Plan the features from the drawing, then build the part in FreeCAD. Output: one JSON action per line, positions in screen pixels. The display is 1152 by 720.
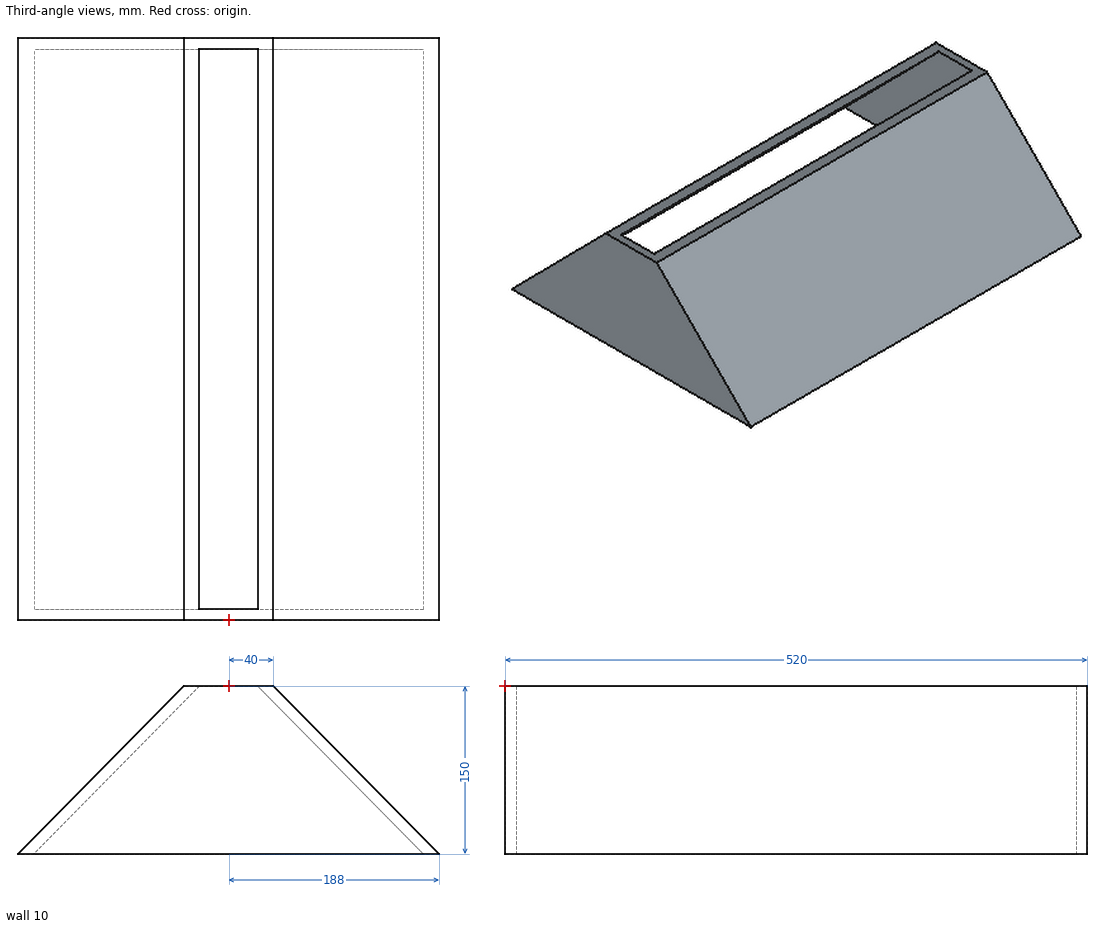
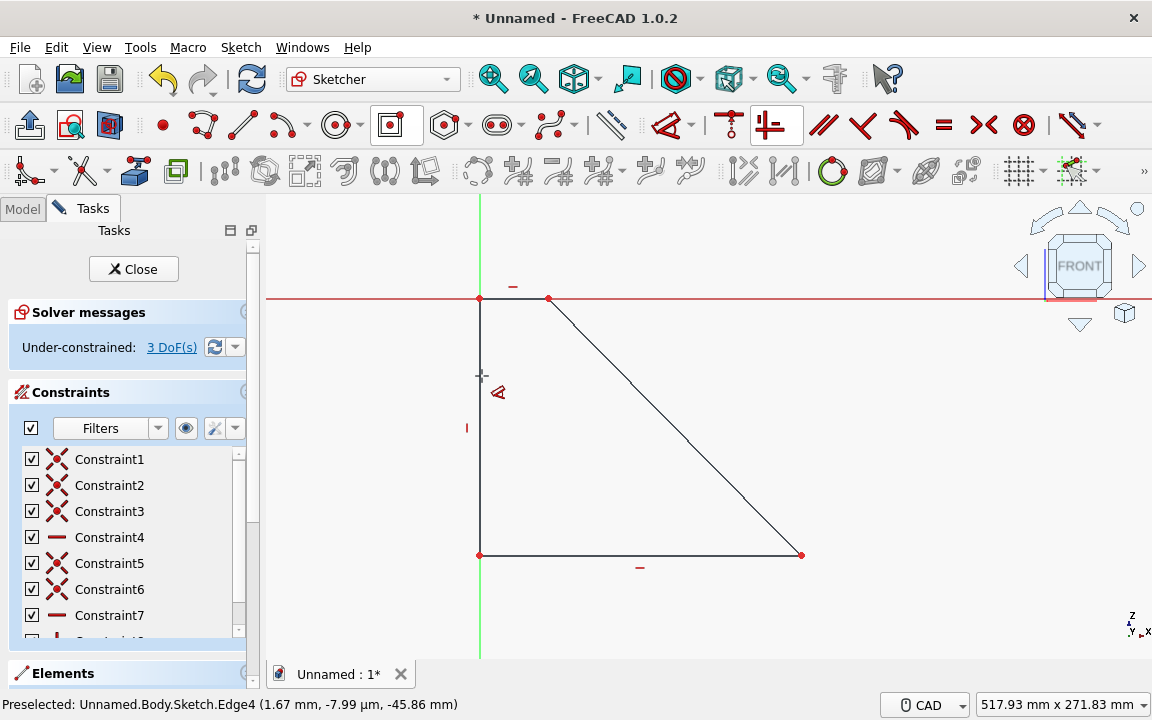
{"action": "left_click", "coordinate": [500, 299]}
{"action": "left_click", "coordinate": [514, 265]}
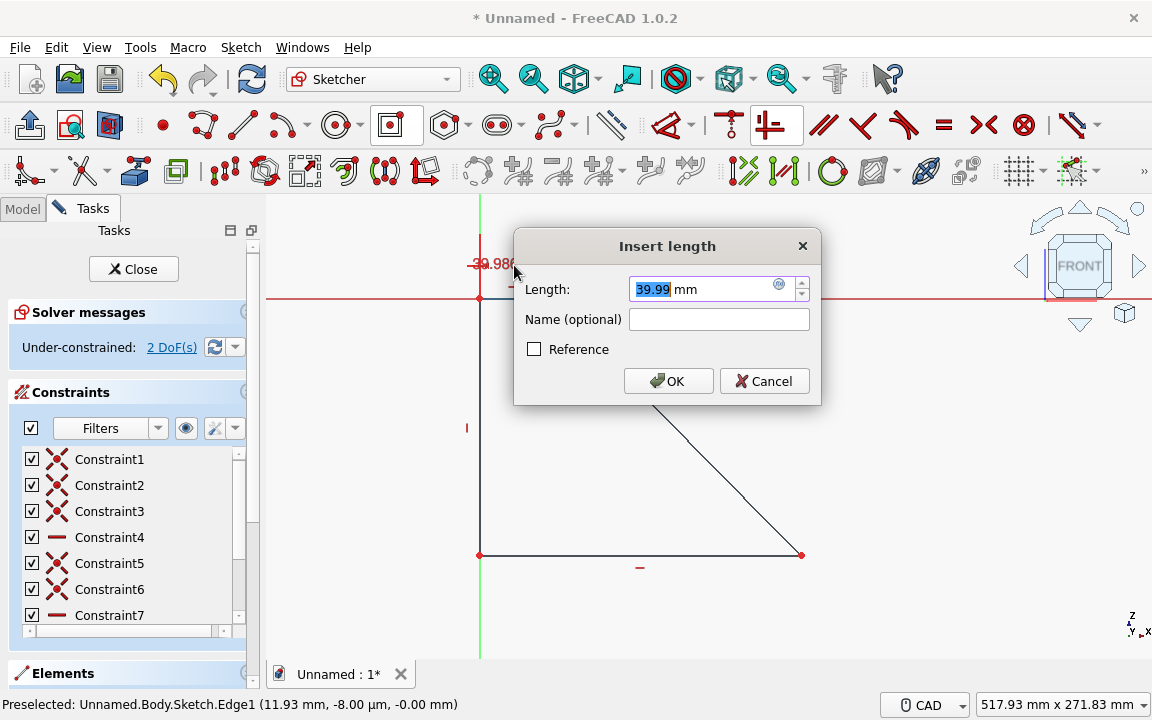
{"action": "type", "text": "40"}
{"action": "key", "text": "Return"}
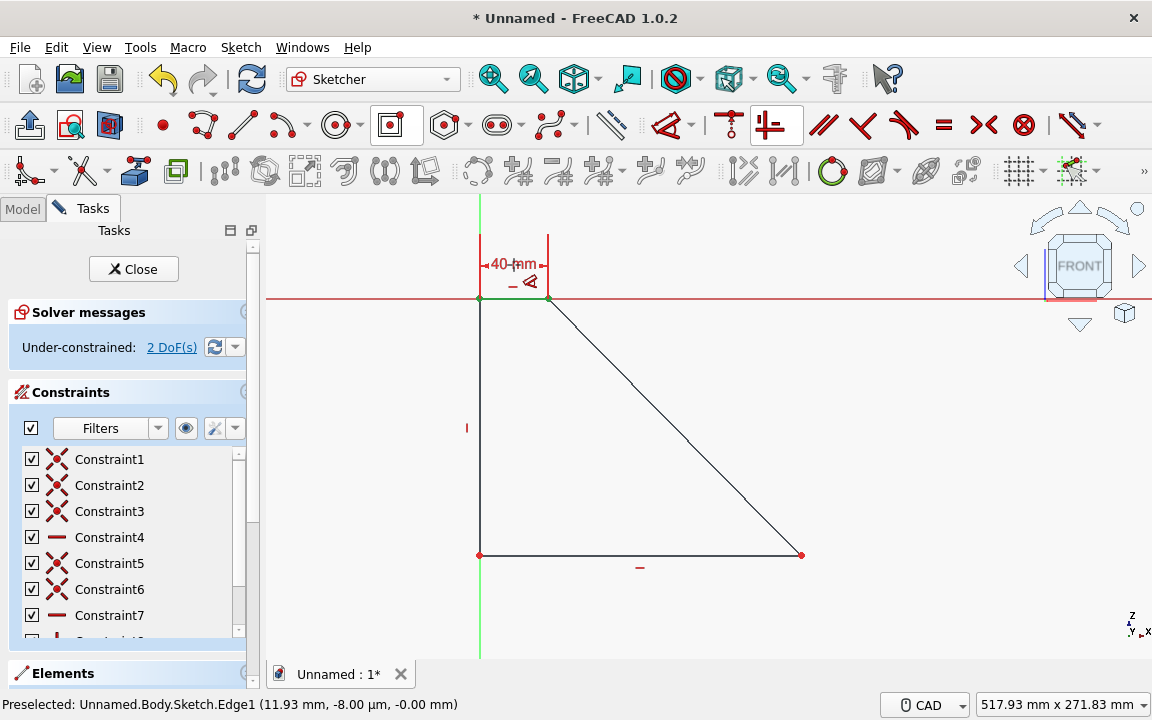
{"action": "left_click", "coordinate": [705, 556]}
{"action": "left_click", "coordinate": [640, 590]}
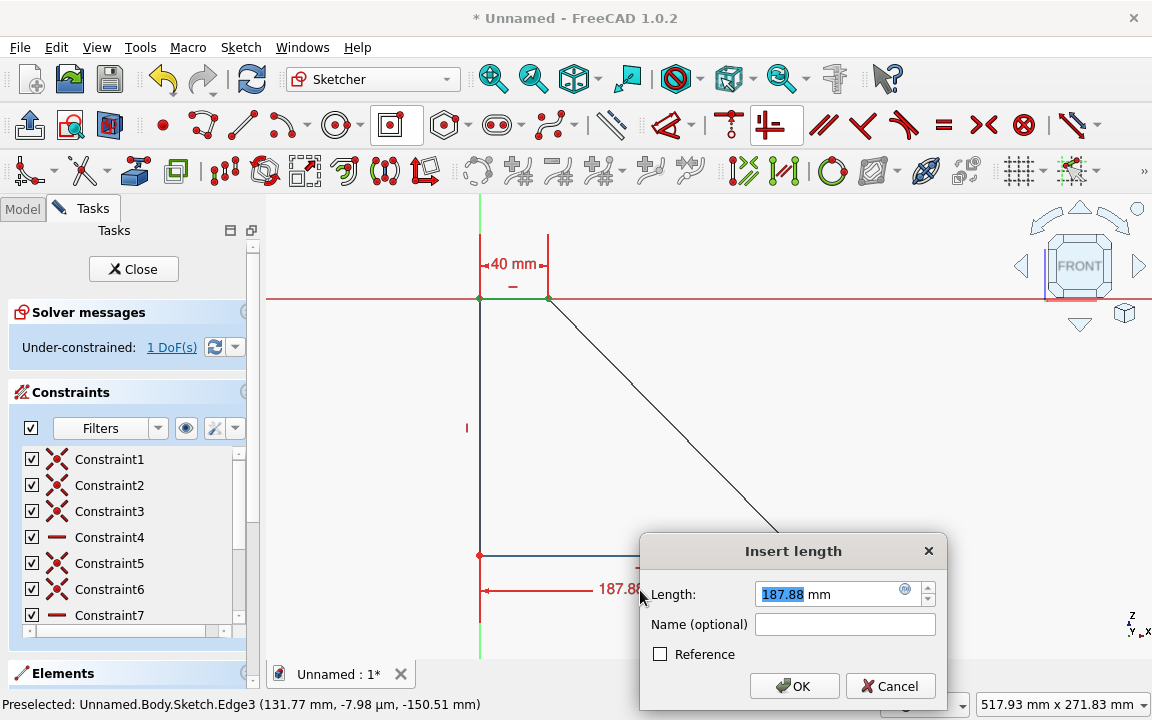
{"action": "type", "text": "188"}
{"action": "key", "text": "Return"}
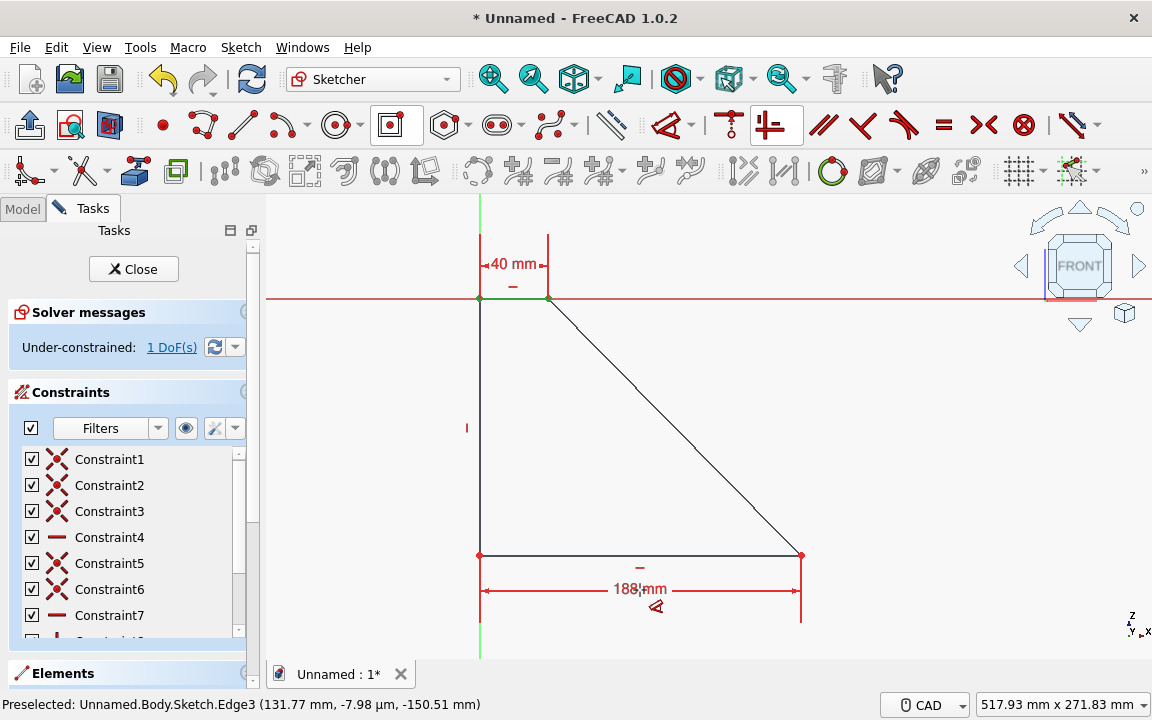
{"action": "left_click", "coordinate": [480, 479]}
{"action": "left_click", "coordinate": [446, 427]}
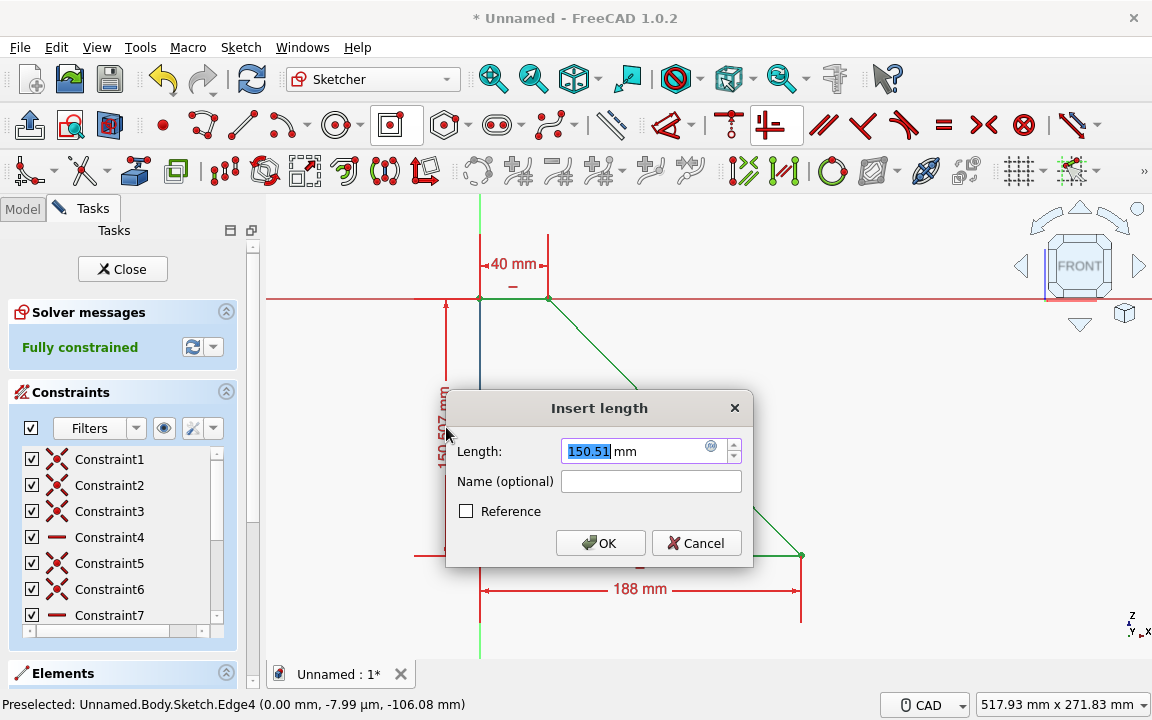
{"action": "type", "text": "150"}
{"action": "key", "text": "Return"}
{"action": "key", "text": "Escape"}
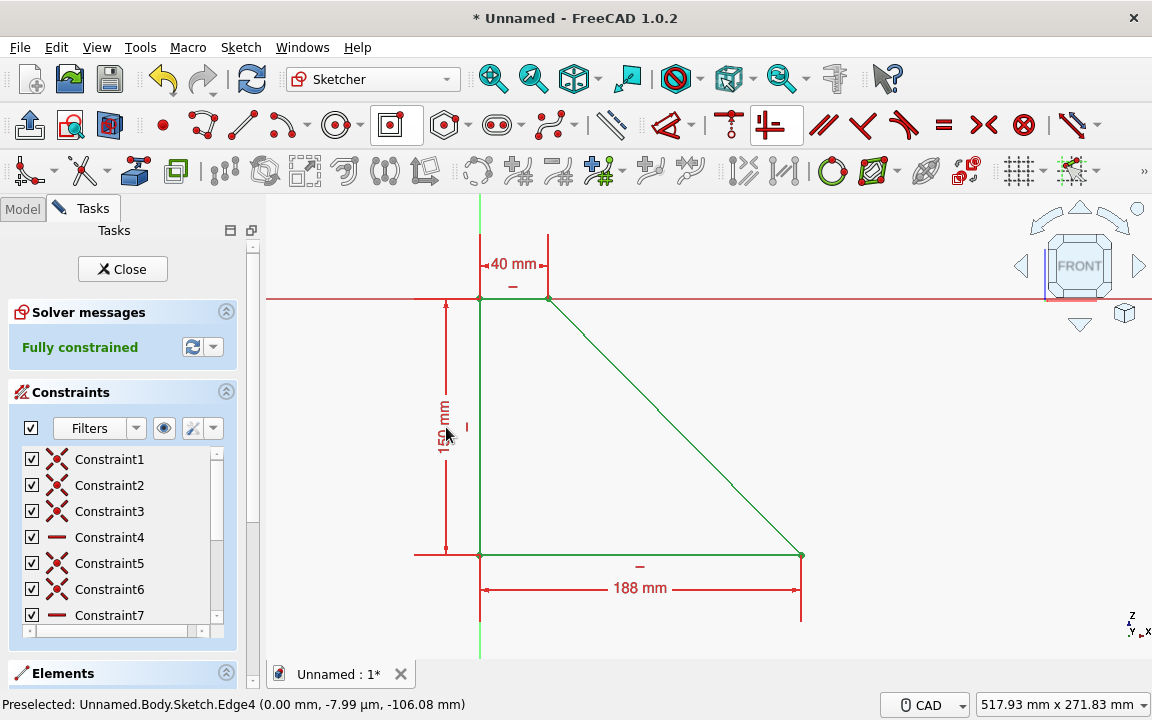
{"action": "left_click", "coordinate": [123, 269]}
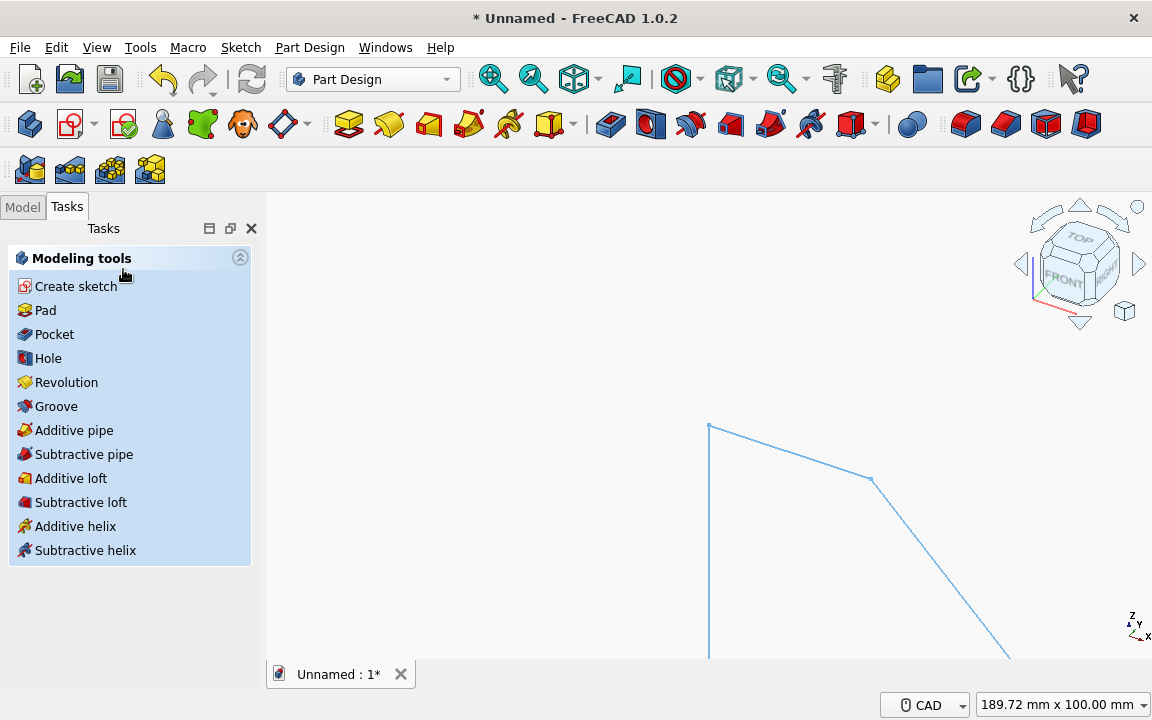
{"action": "left_click", "coordinate": [350, 124]}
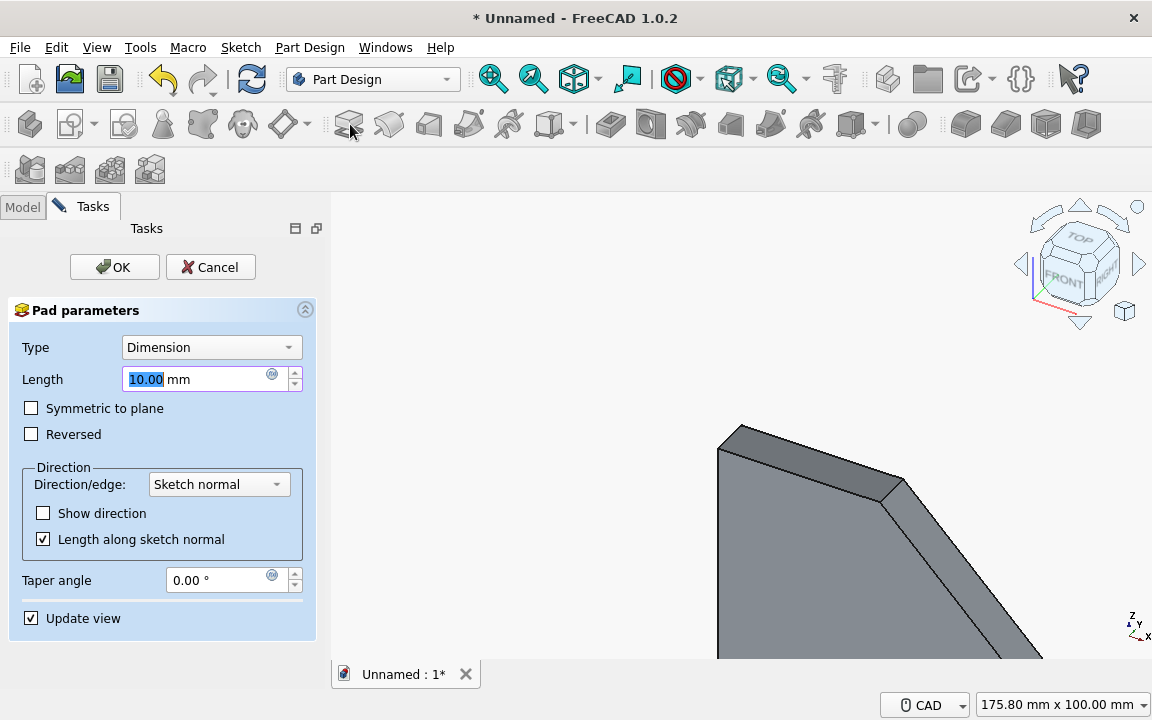
{"action": "type", "text": "520"}
{"action": "key", "text": "Tab"}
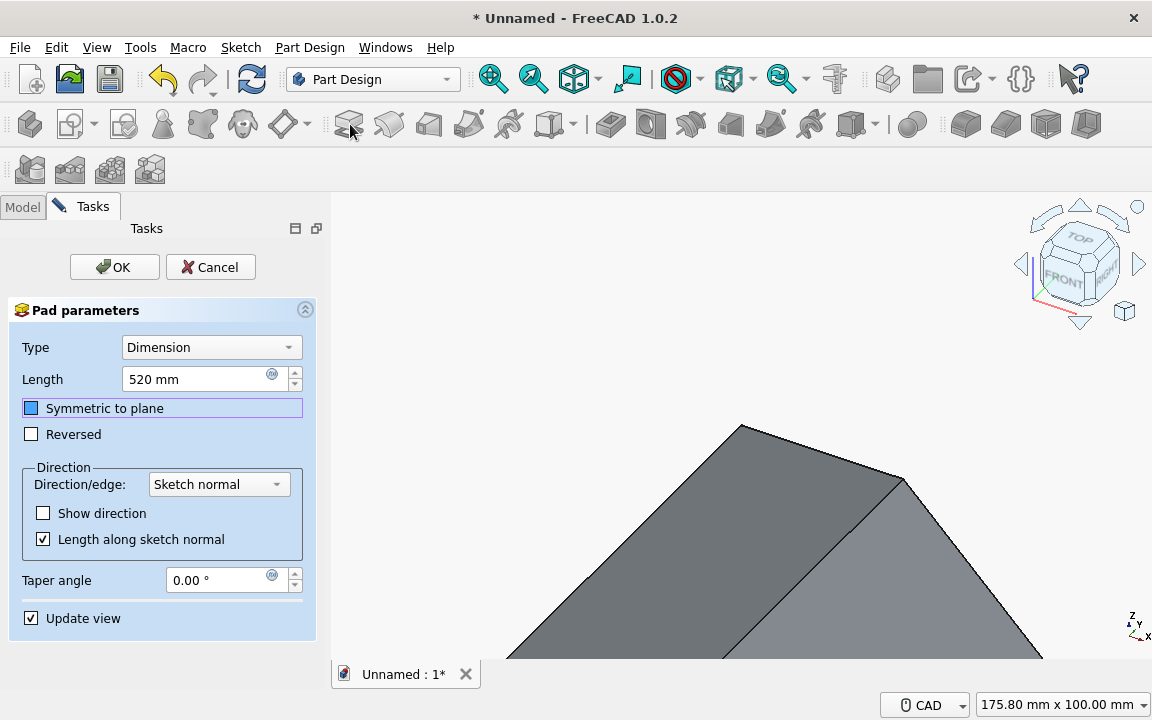
{"action": "left_click", "coordinate": [30, 434]}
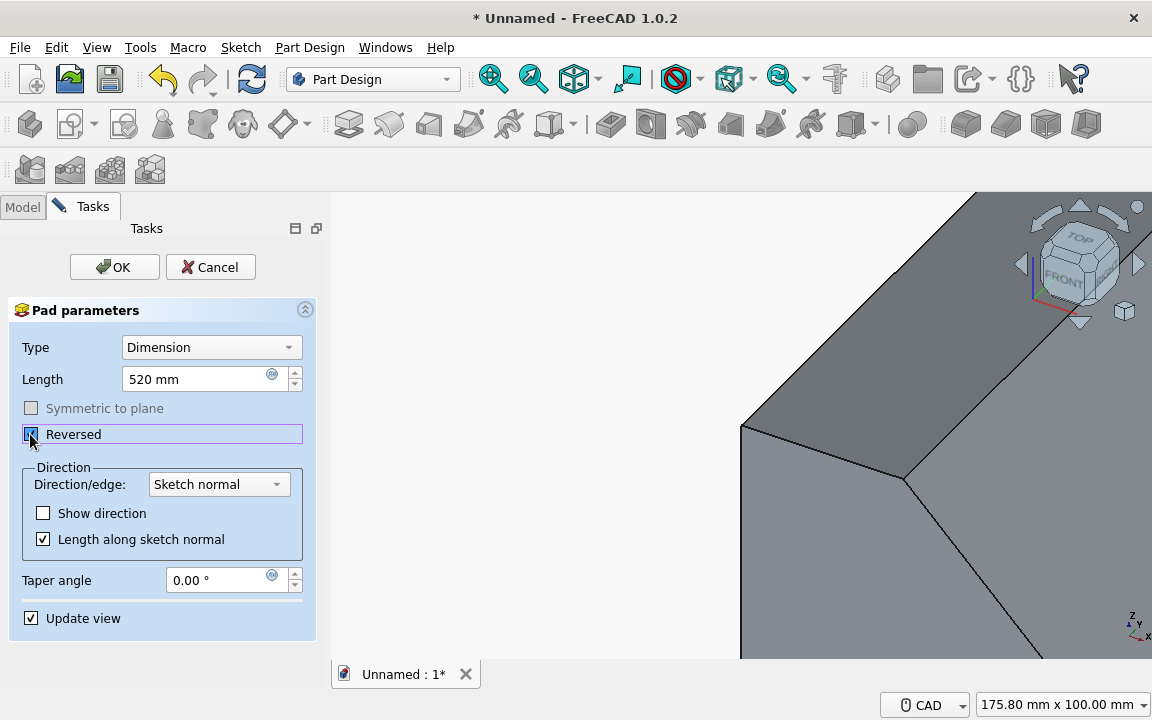
{"action": "left_click", "coordinate": [115, 267]}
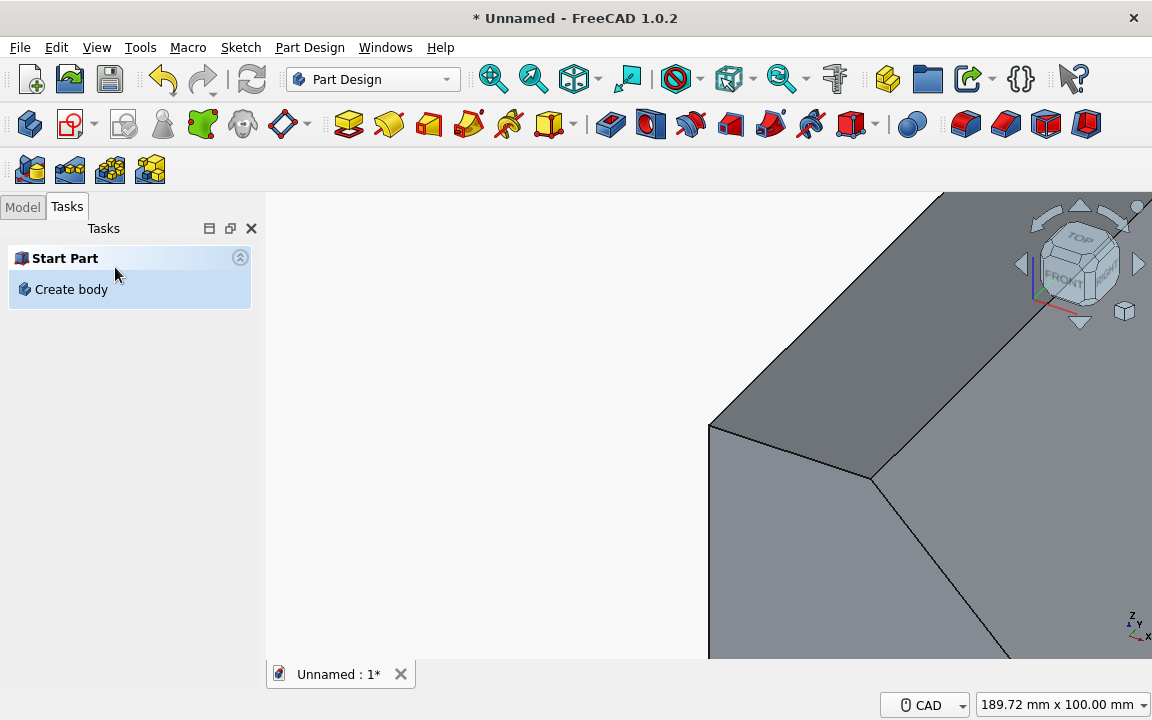
{"action": "left_click", "coordinate": [494, 80]}